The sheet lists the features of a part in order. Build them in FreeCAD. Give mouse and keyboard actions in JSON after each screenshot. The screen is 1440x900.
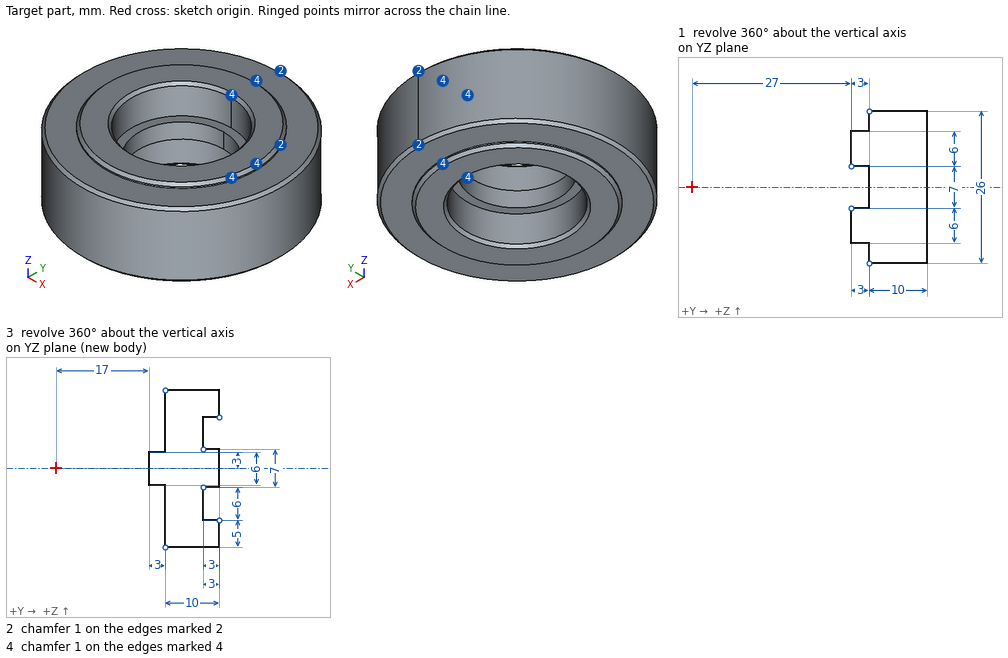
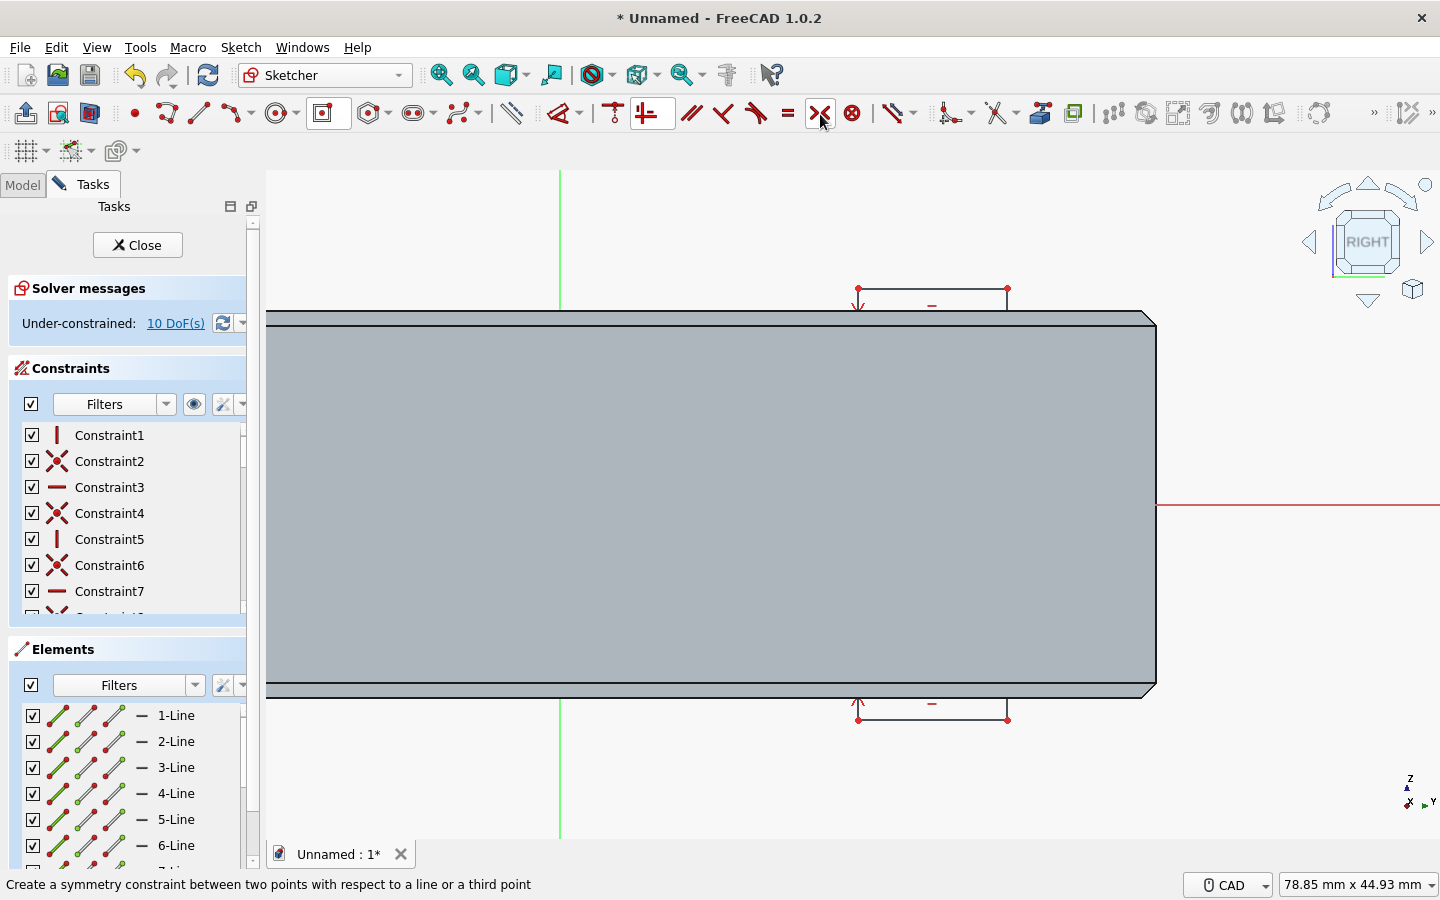
{"action": "left_click", "coordinate": [558, 114]}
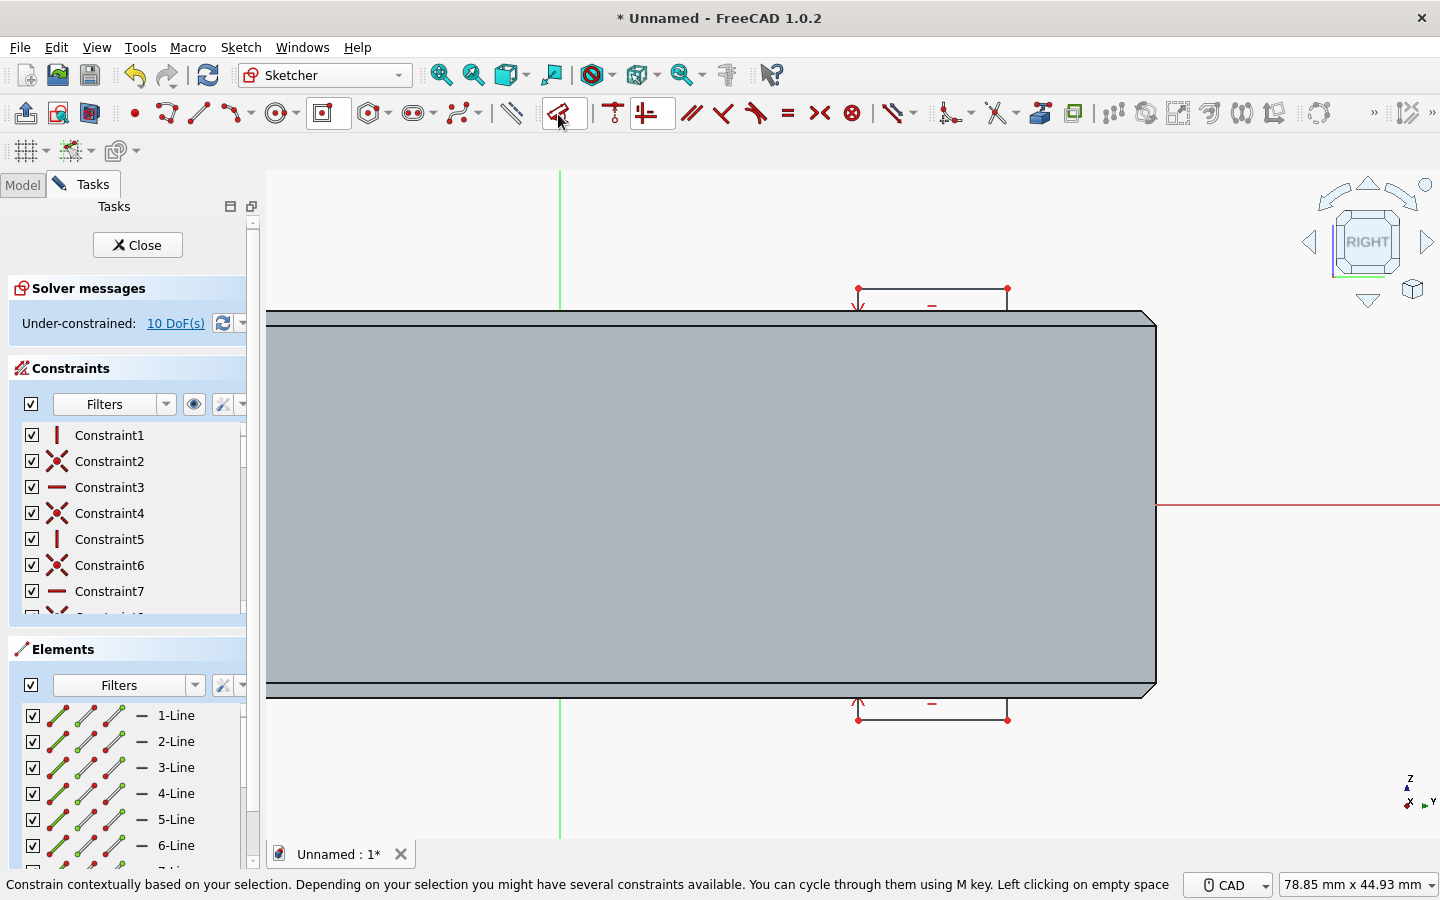
{"action": "left_click", "coordinate": [814, 488]}
{"action": "left_click", "coordinate": [848, 485]}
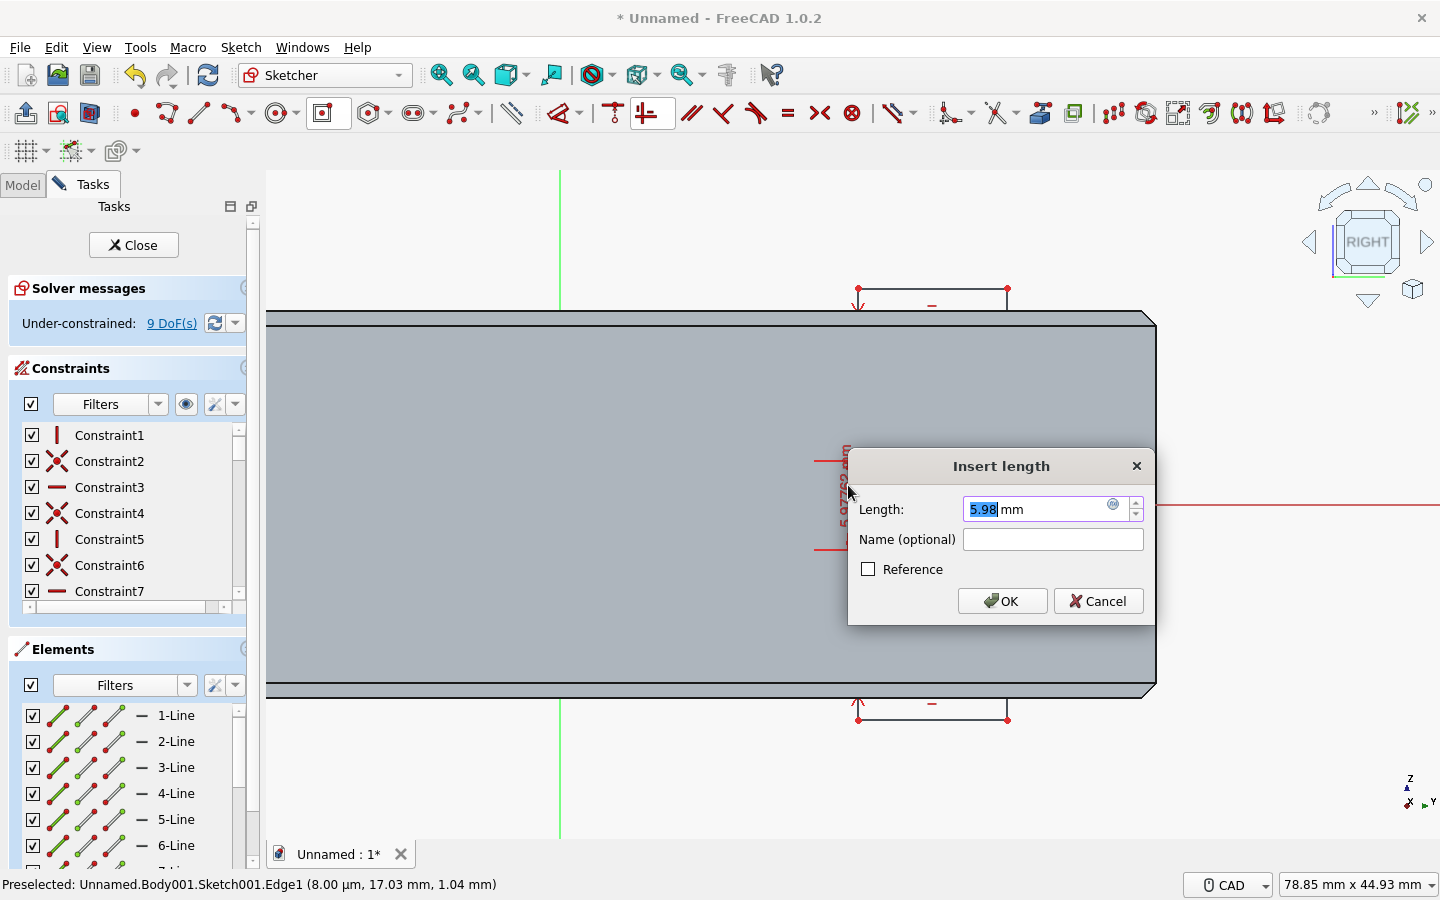
{"action": "type", "text": "6"}
{"action": "key", "text": "Return"}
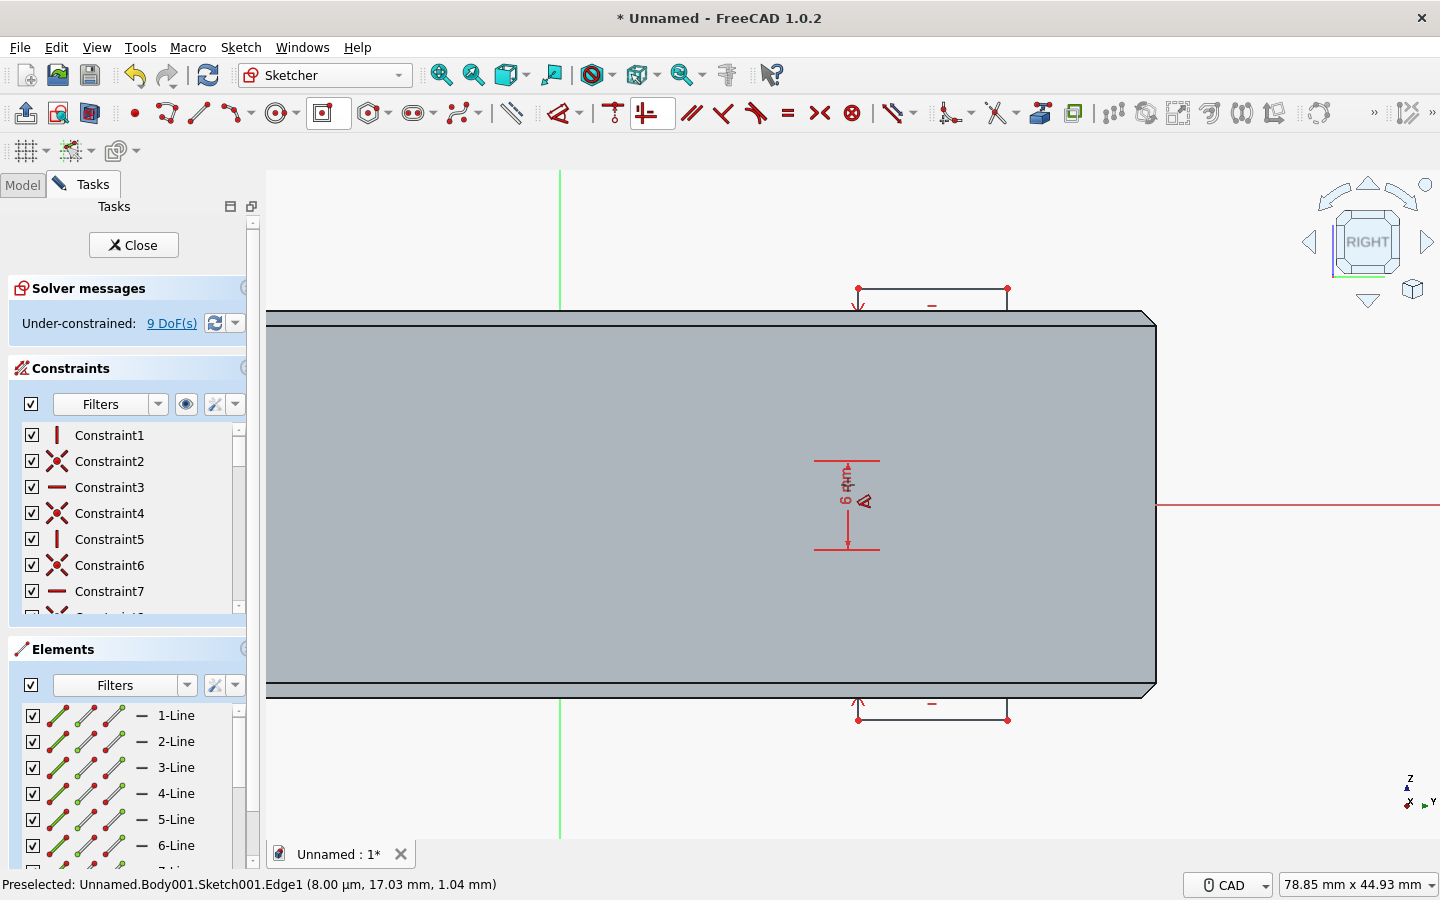
{"action": "left_click", "coordinate": [827, 550]}
{"action": "left_click", "coordinate": [836, 584]}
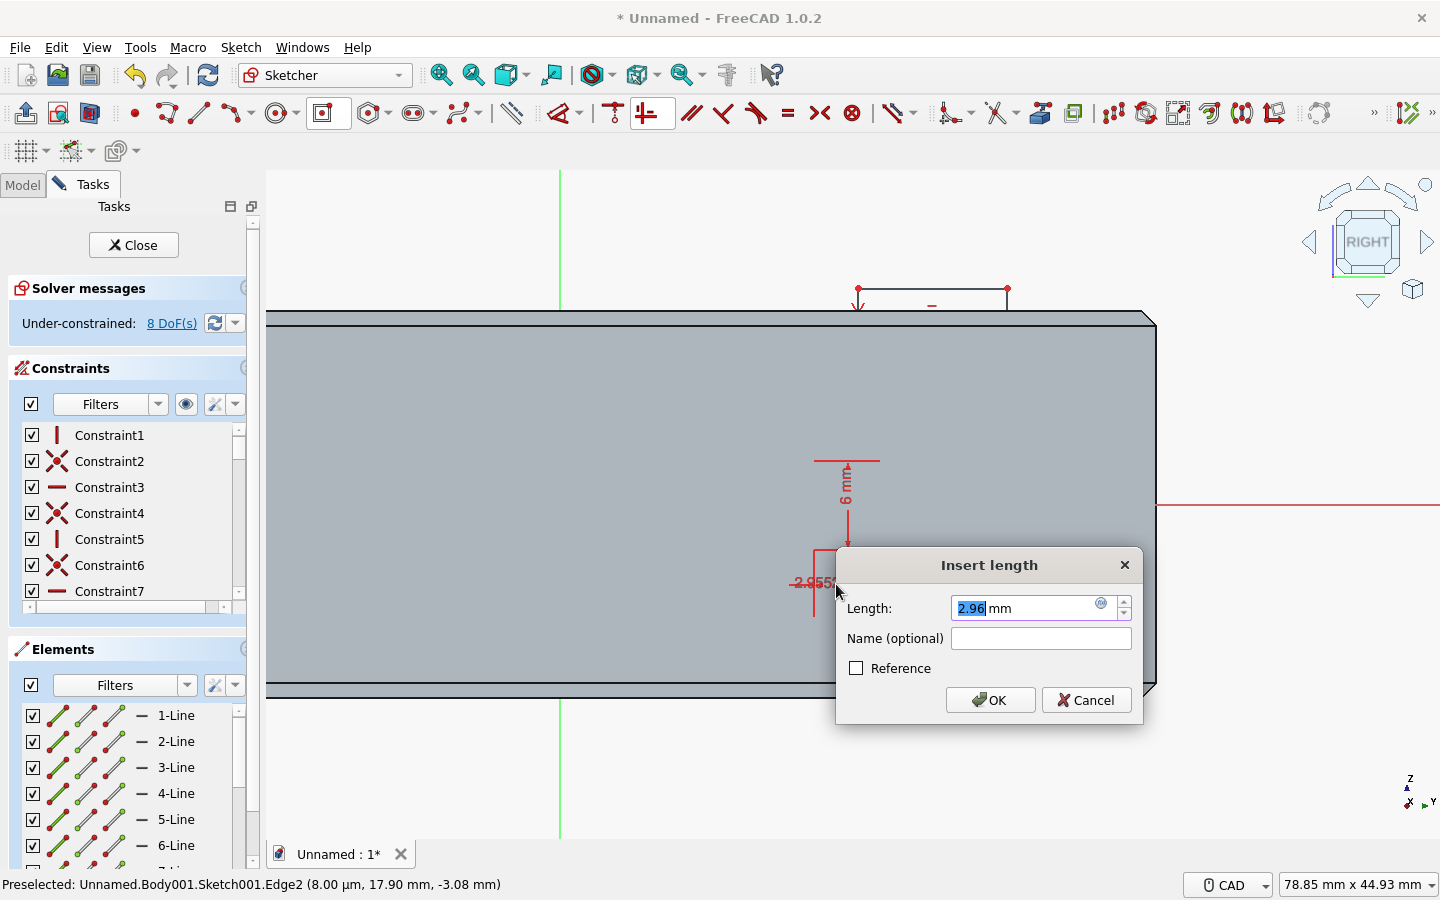
{"action": "type", "text": "3"}
{"action": "key", "text": "Return"}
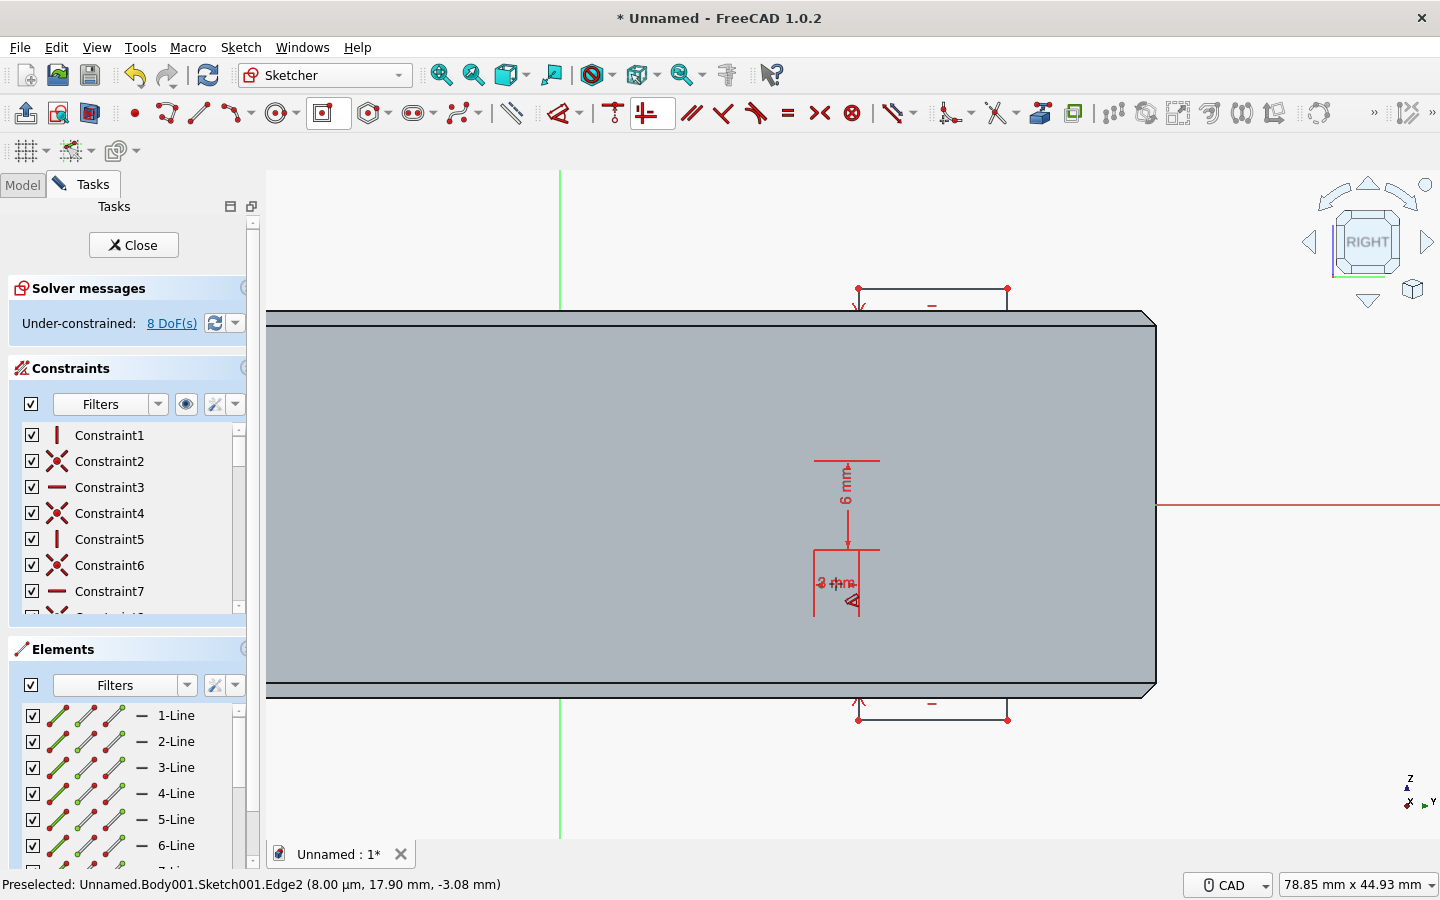
{"action": "left_click", "coordinate": [1007, 698]}
{"action": "left_click", "coordinate": [1041, 683]}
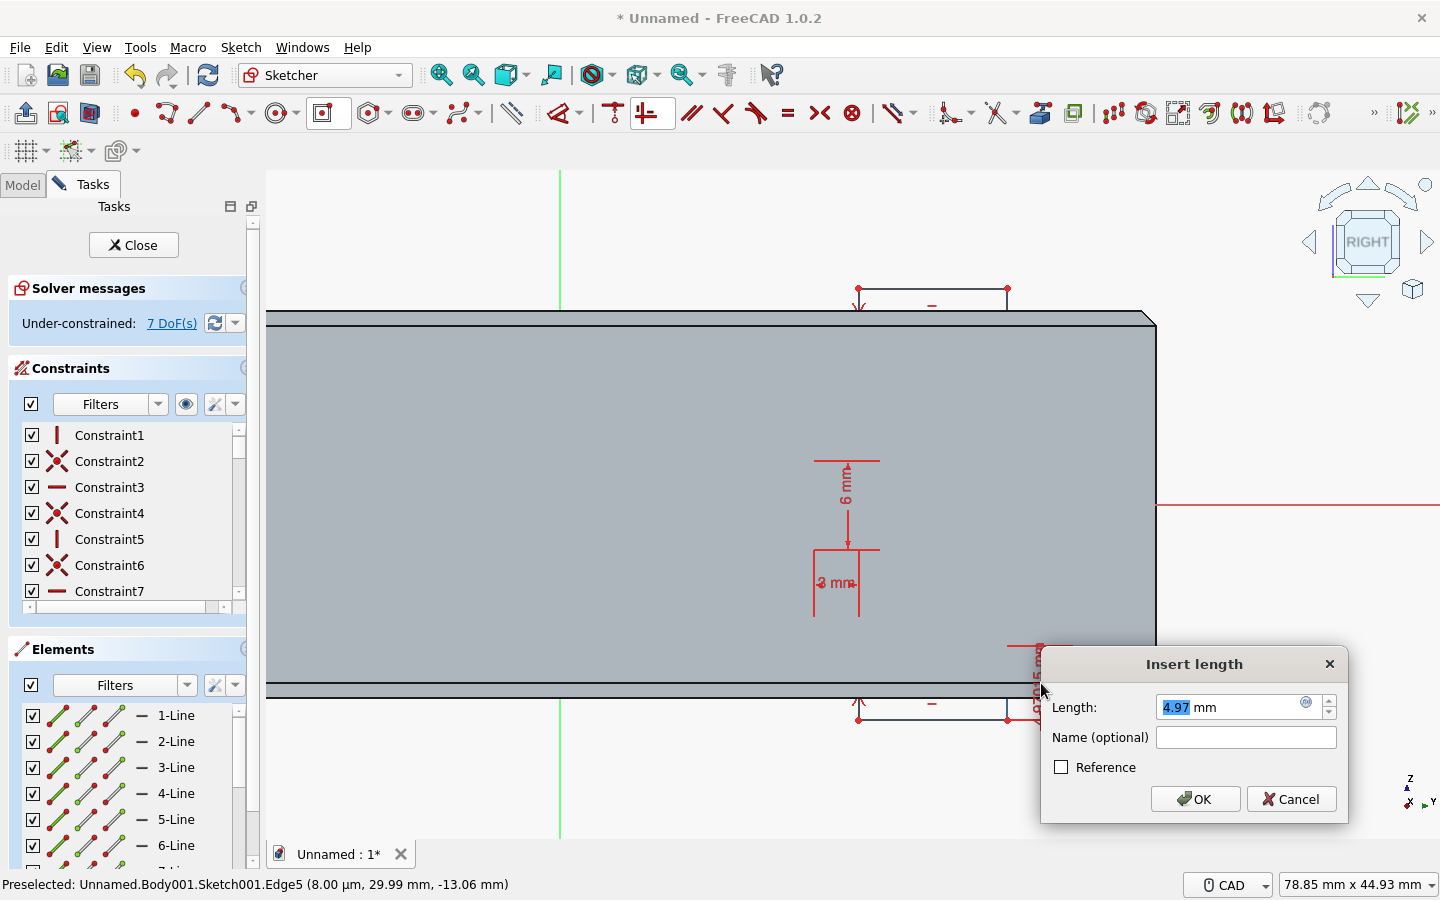
{"action": "type", "text": "5"}
{"action": "key", "text": "Return"}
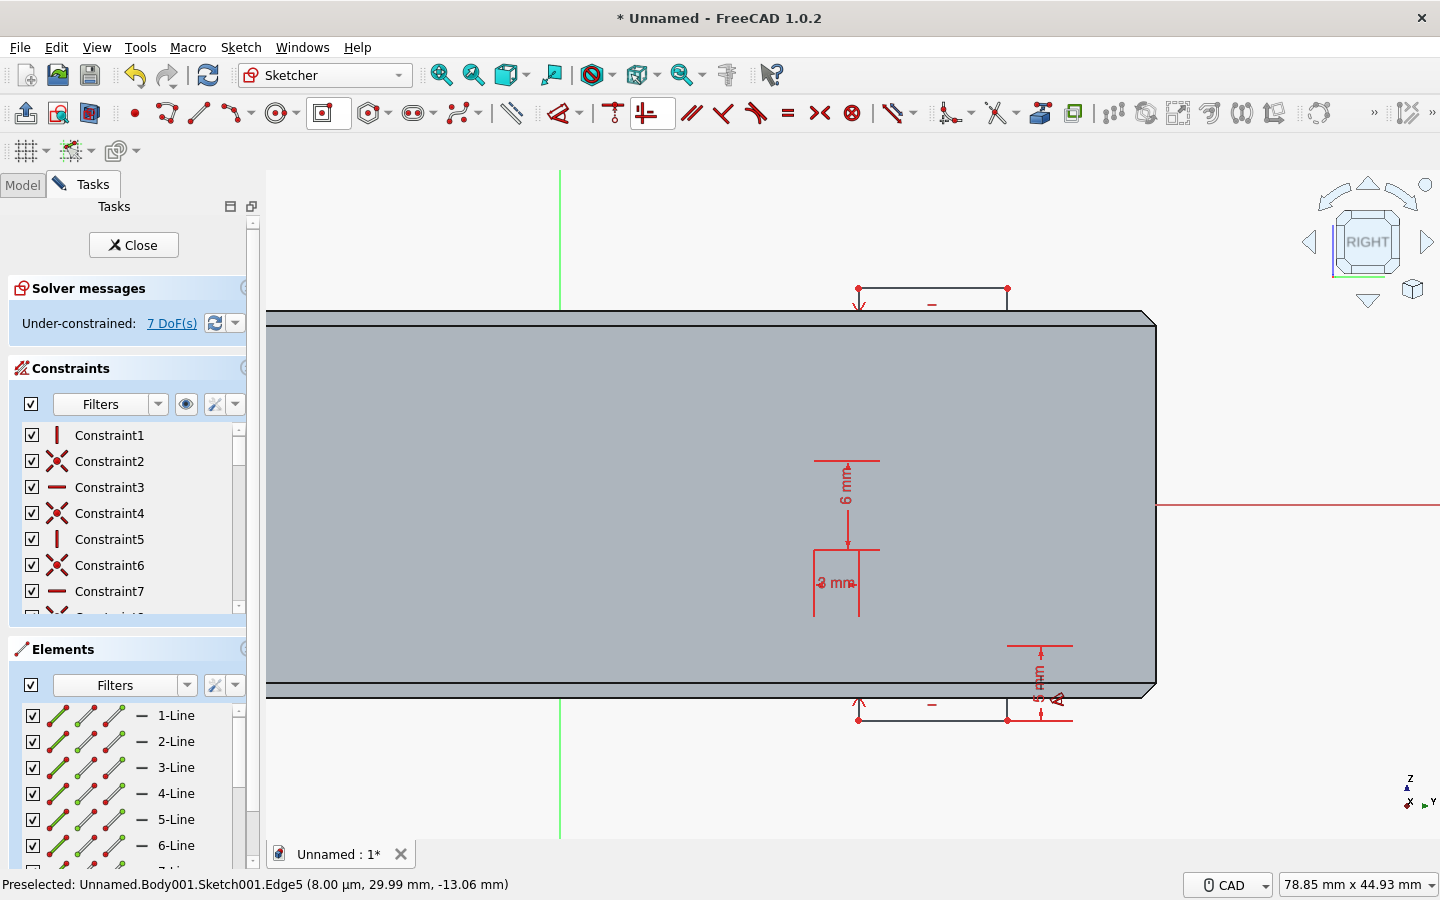
{"action": "left_click", "coordinate": [993, 646]}
{"action": "left_click", "coordinate": [969, 680]}